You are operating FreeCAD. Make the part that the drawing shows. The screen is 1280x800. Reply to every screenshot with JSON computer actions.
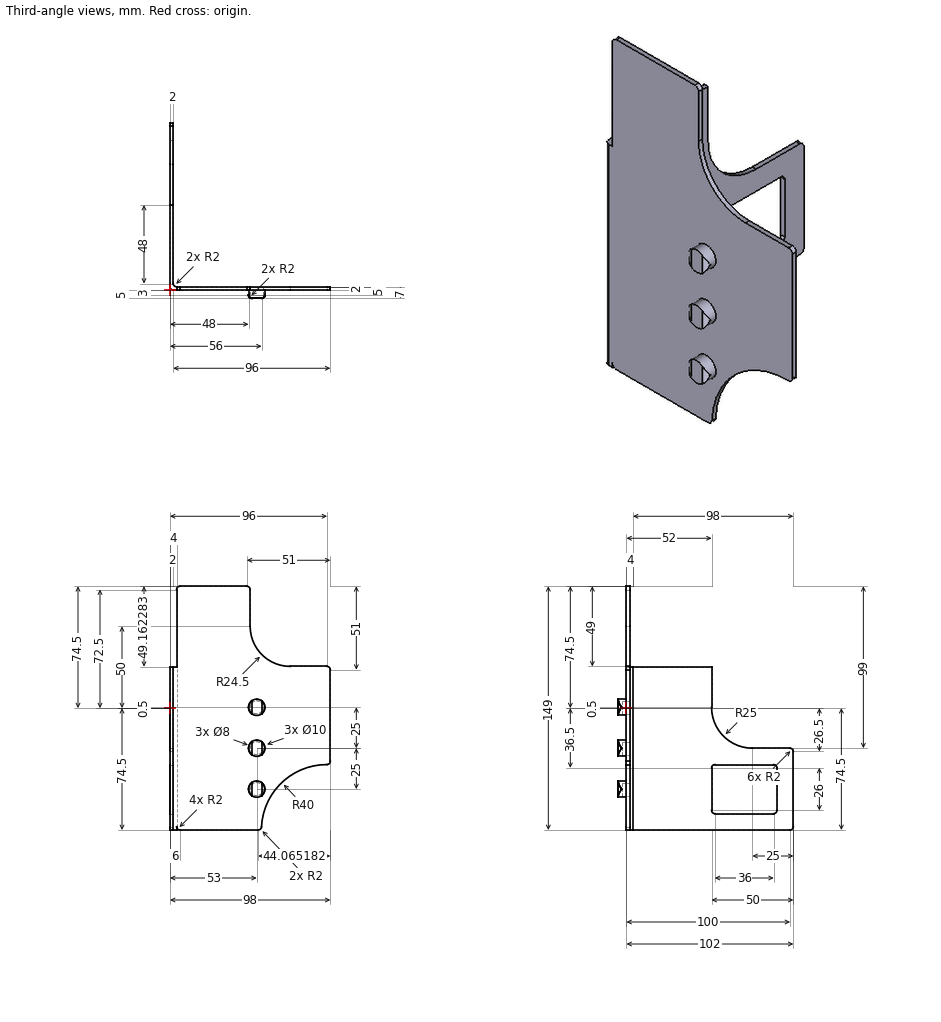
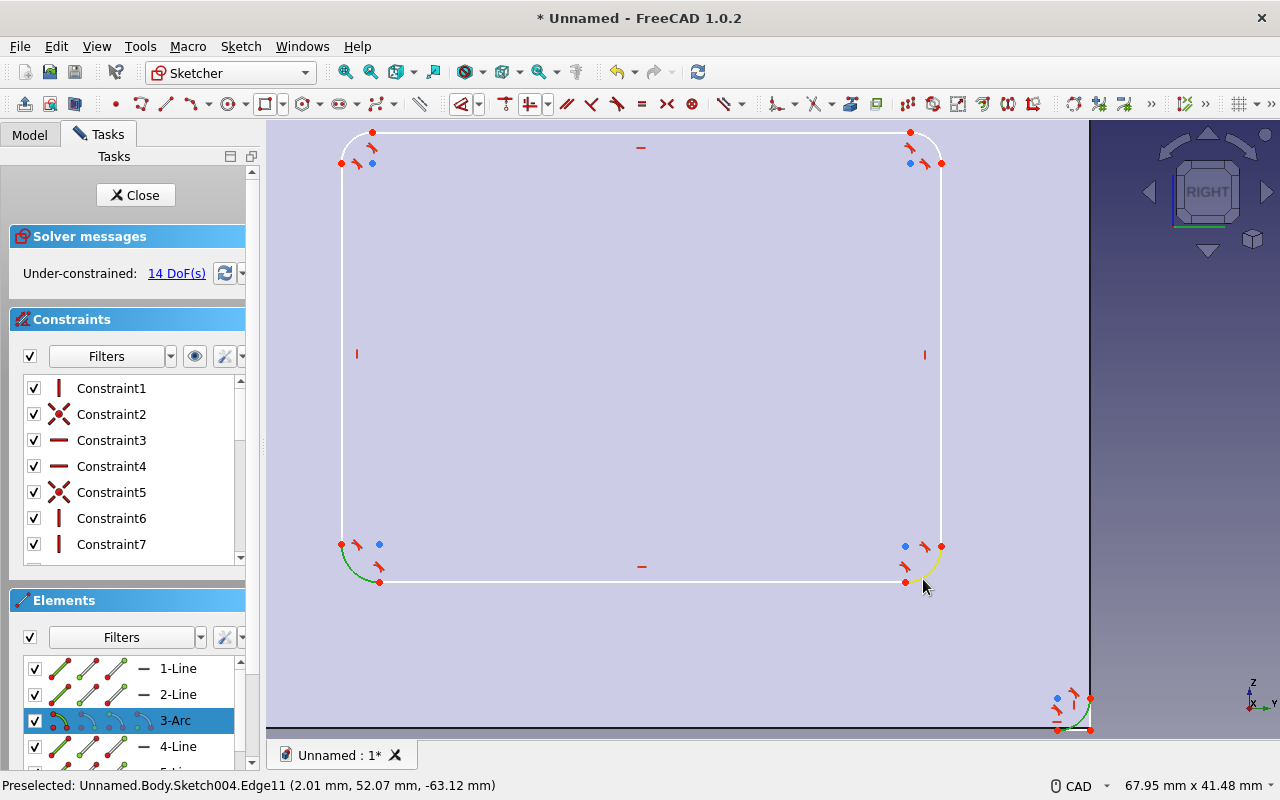
{"action": "left_click", "coordinate": [922, 579]}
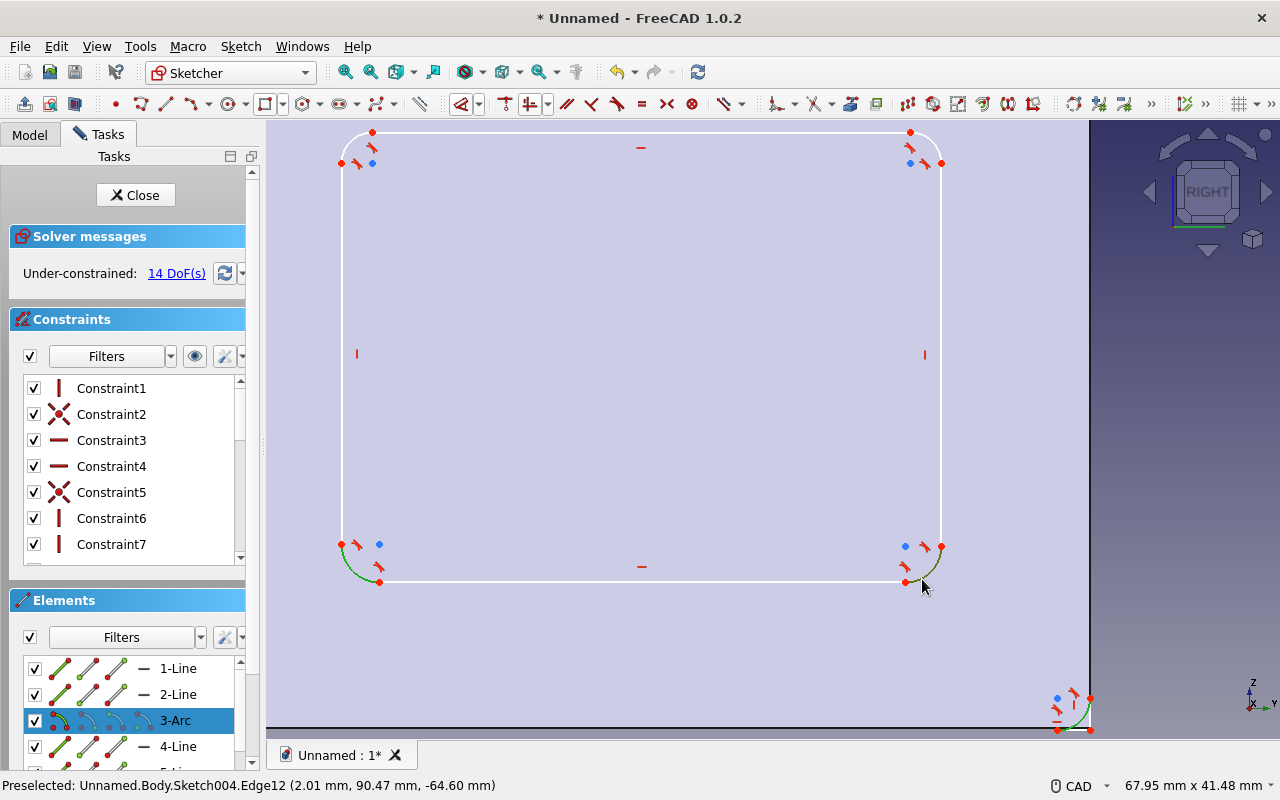
{"action": "left_click", "coordinate": [938, 149]}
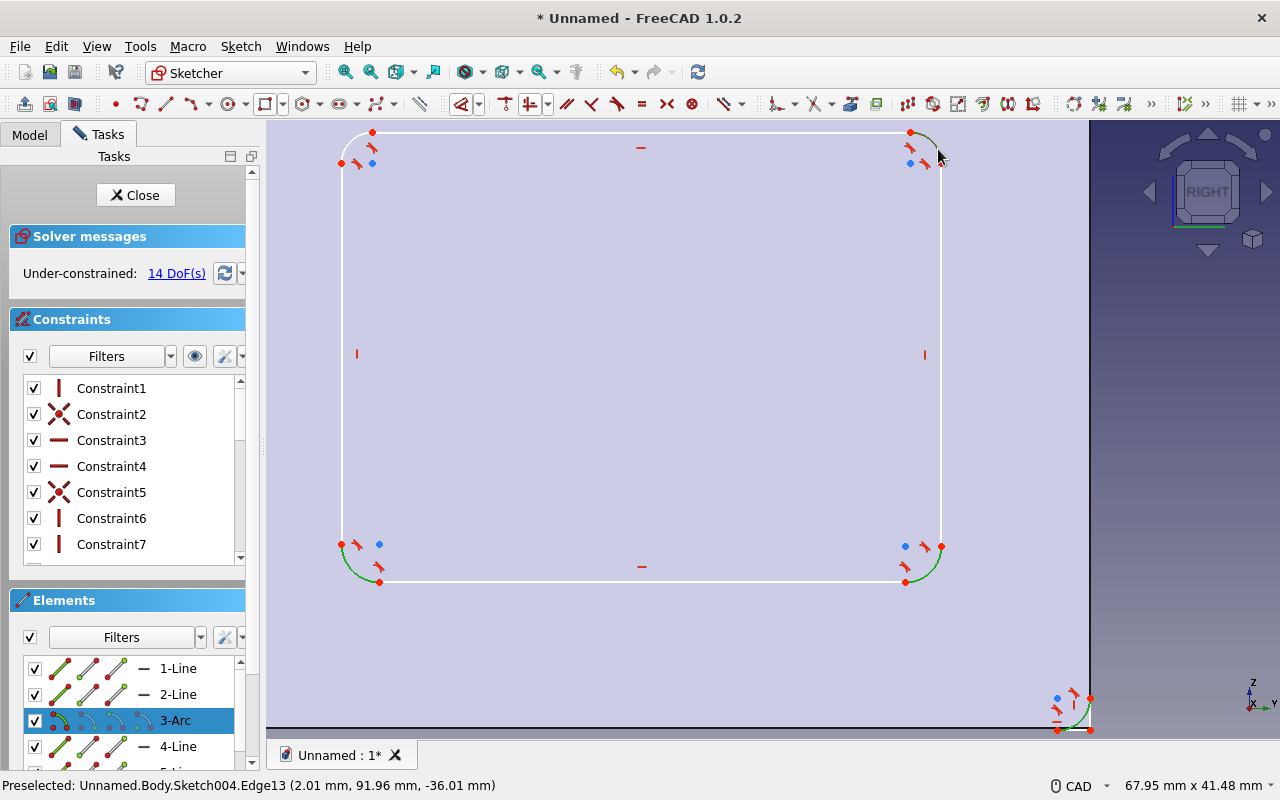
{"action": "left_click", "coordinate": [345, 149]}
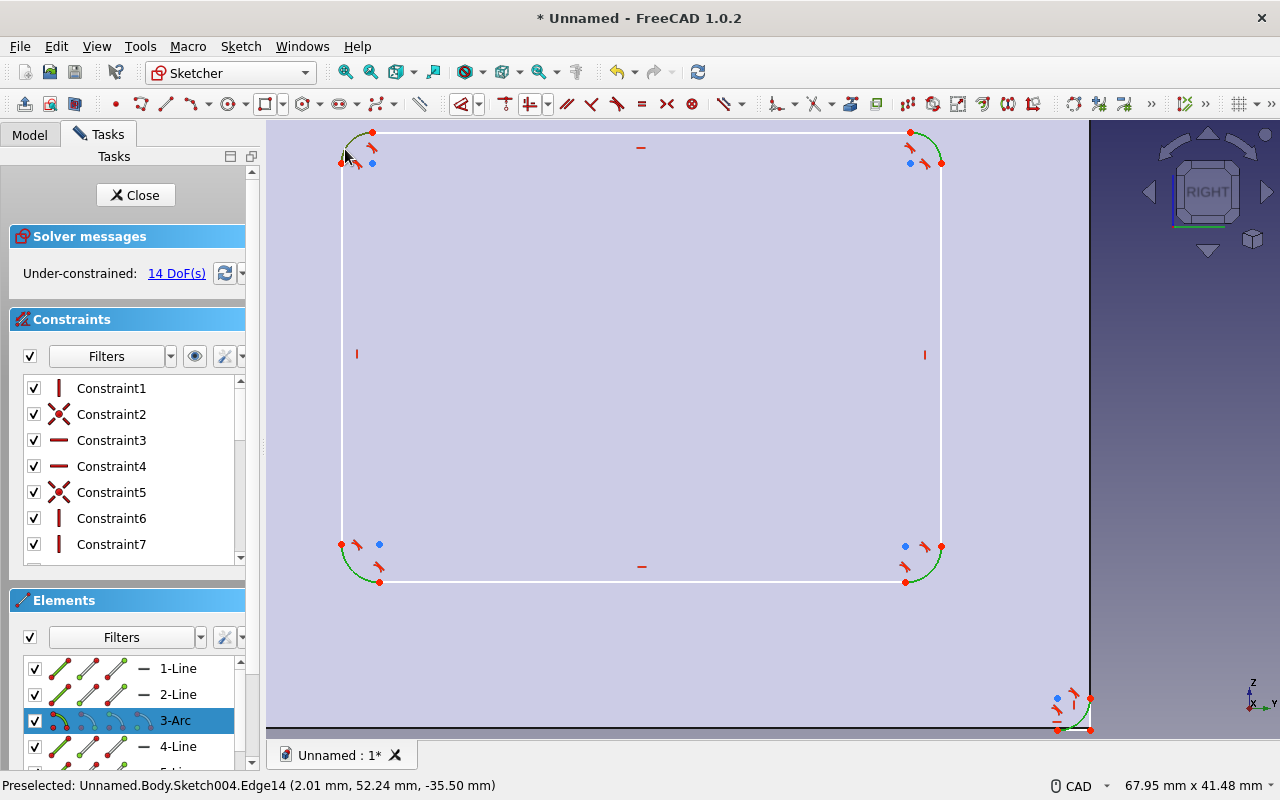
{"action": "key", "text": "e"}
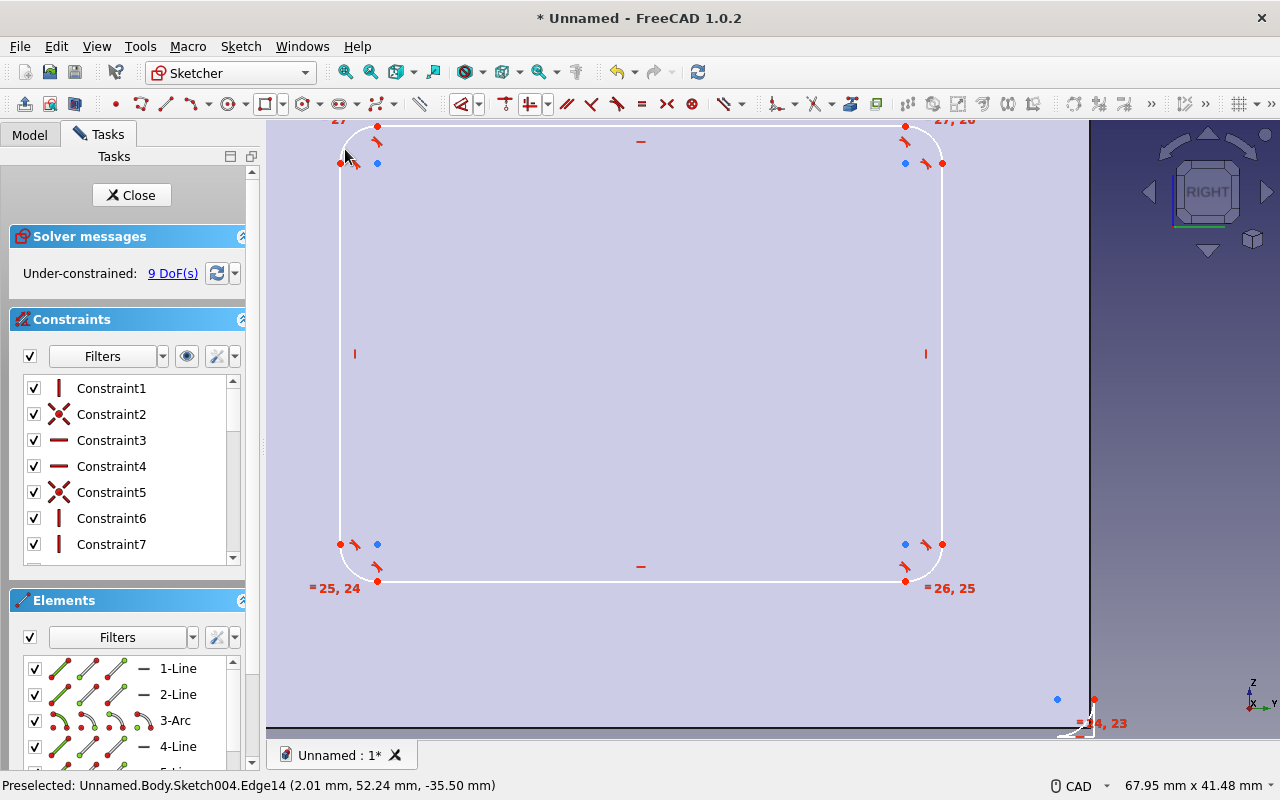
{"action": "scroll", "coordinate": [923, 579], "scroll_direction": "down", "scroll_amount": 5}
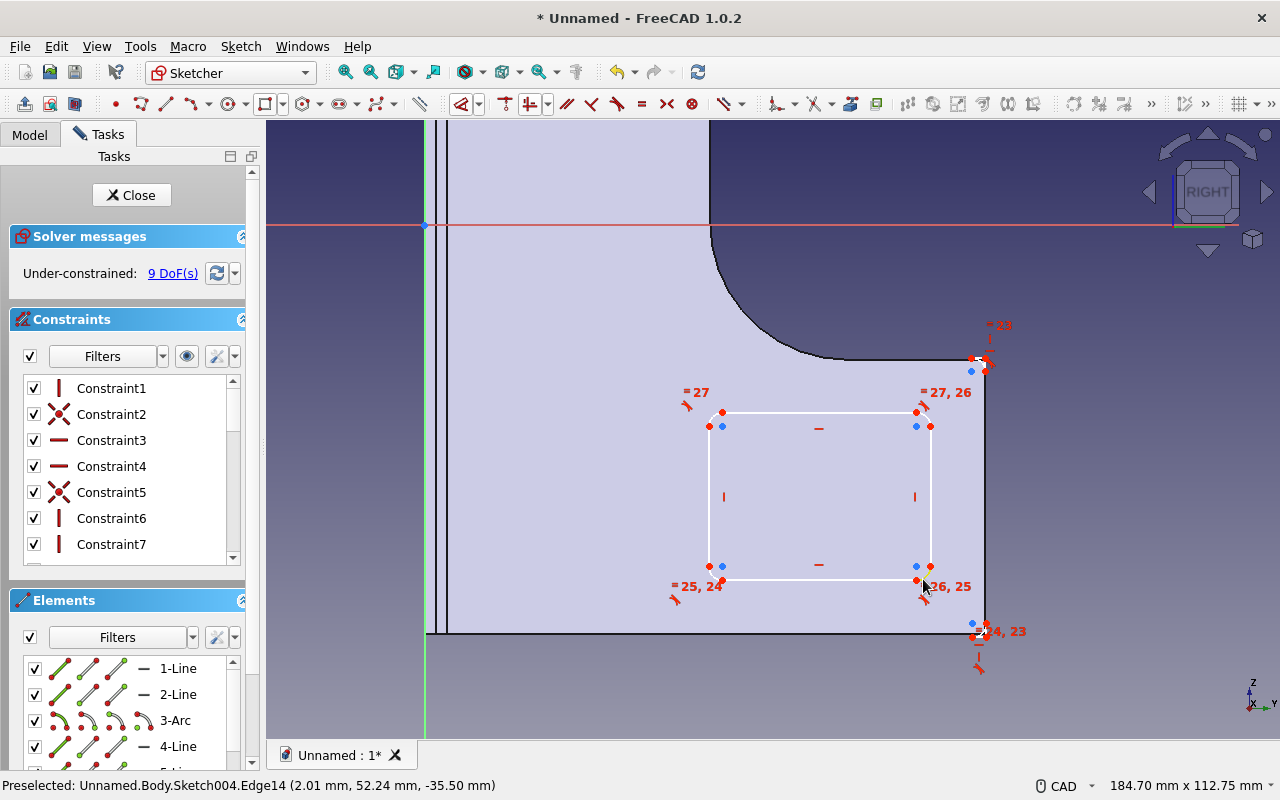
{"action": "scroll", "coordinate": [981, 362], "scroll_direction": "up", "scroll_amount": 7}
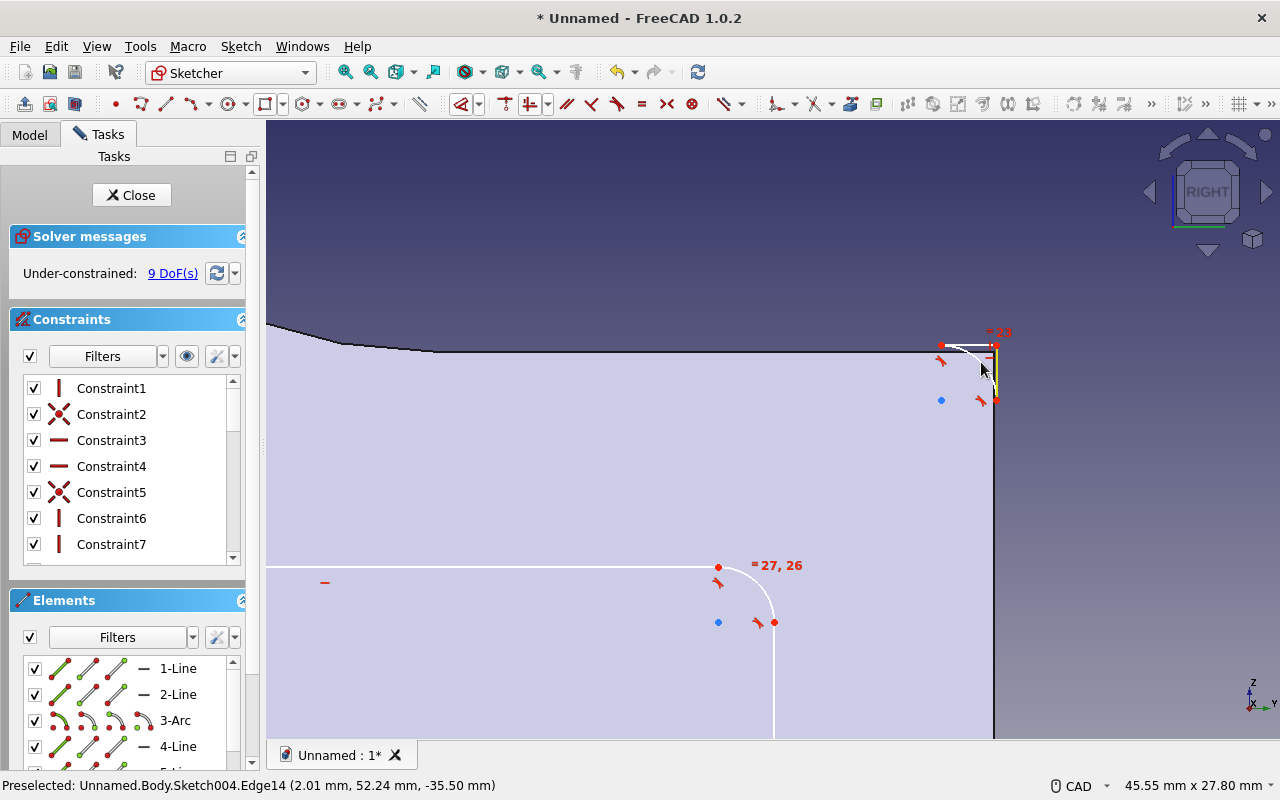
{"action": "left_click", "coordinate": [980, 362]}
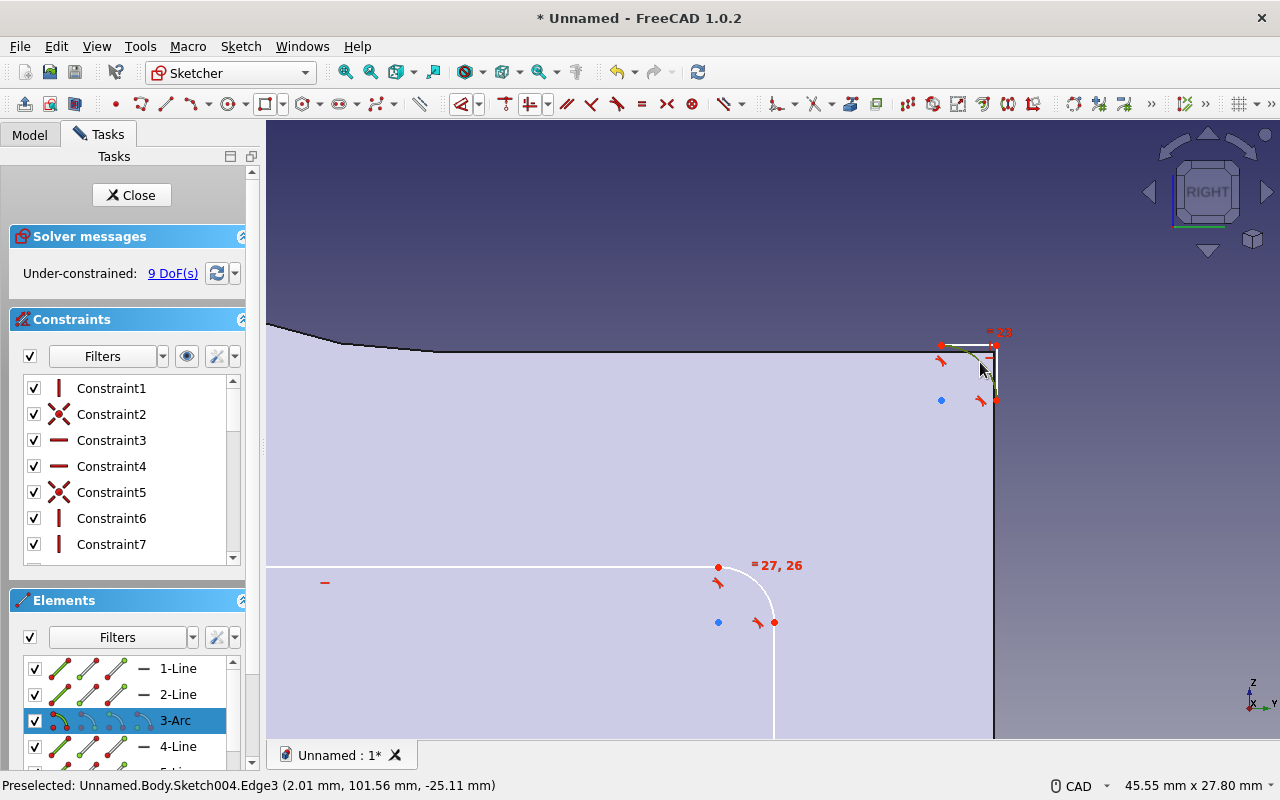
{"action": "key", "text": "k r"}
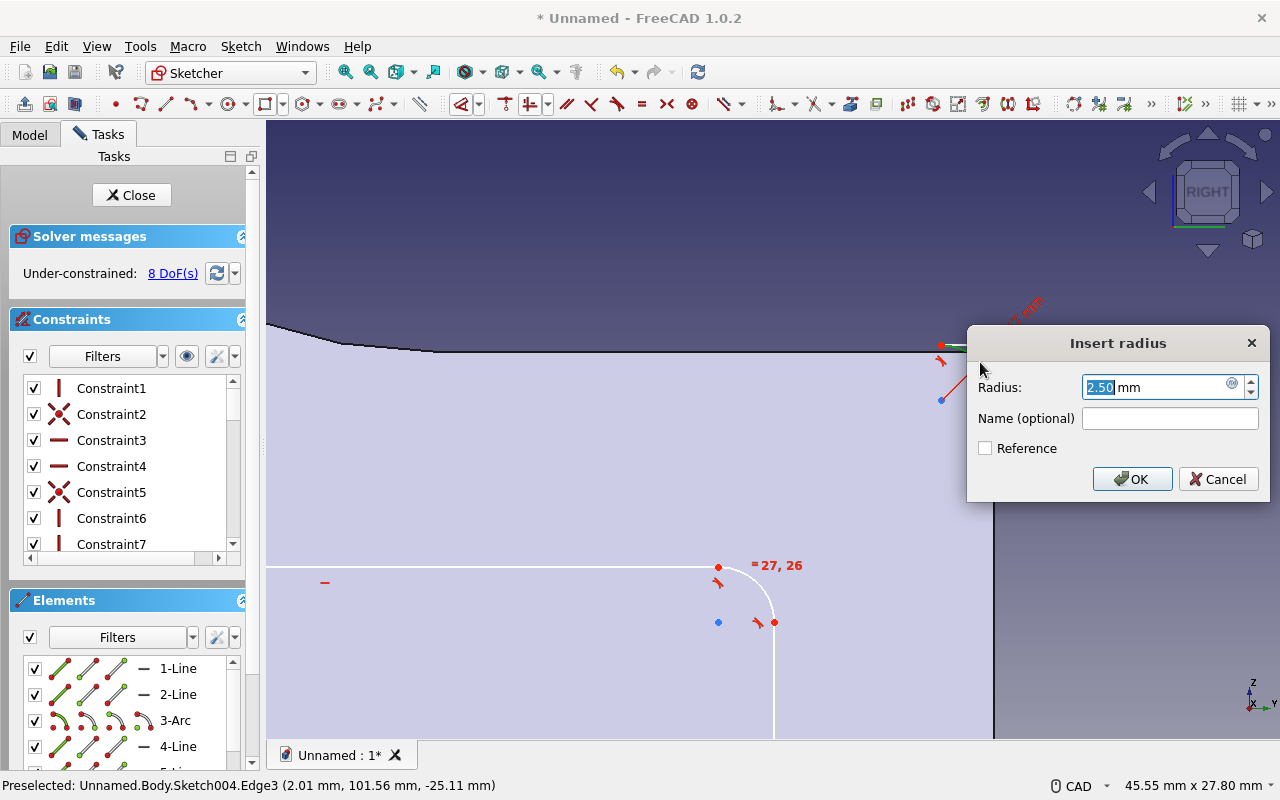
{"action": "type", "text": "2"}
{"action": "key", "text": "Return"}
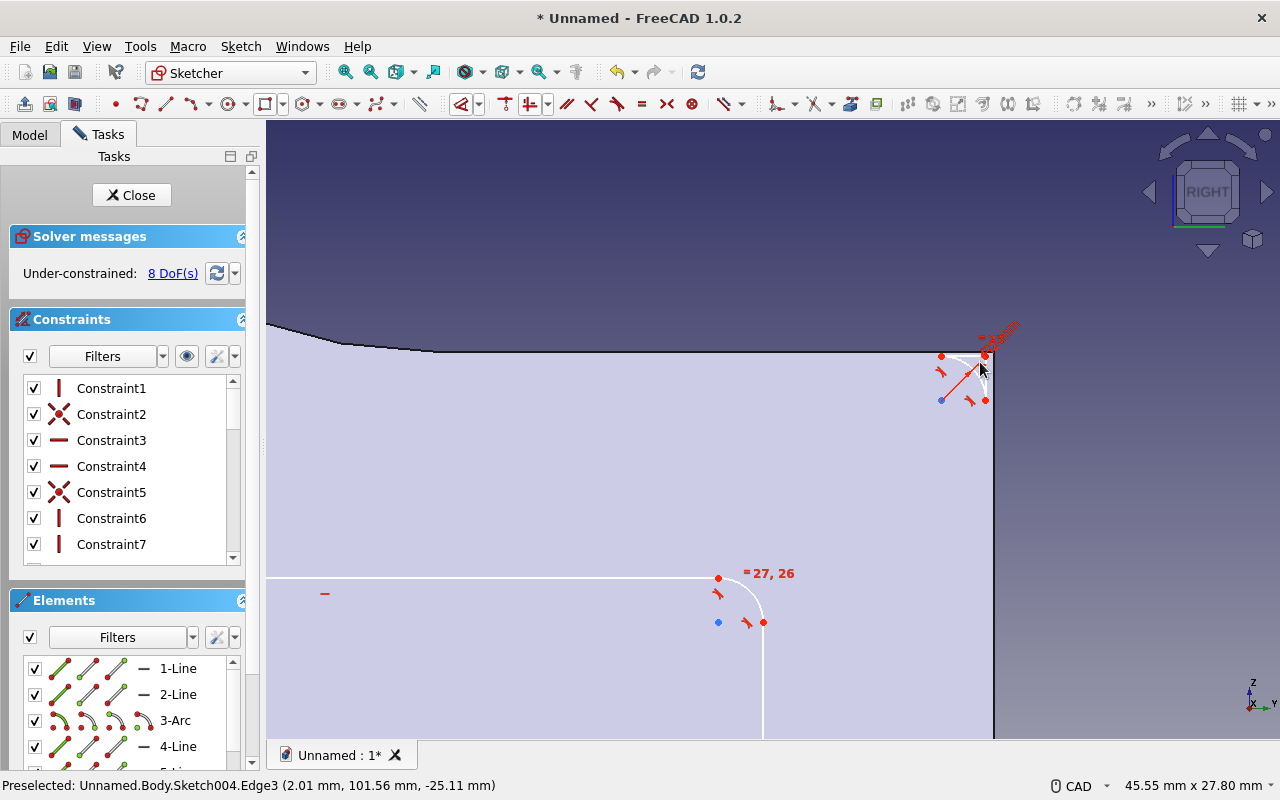
{"action": "scroll", "coordinate": [981, 362], "scroll_direction": "down", "scroll_amount": 7}